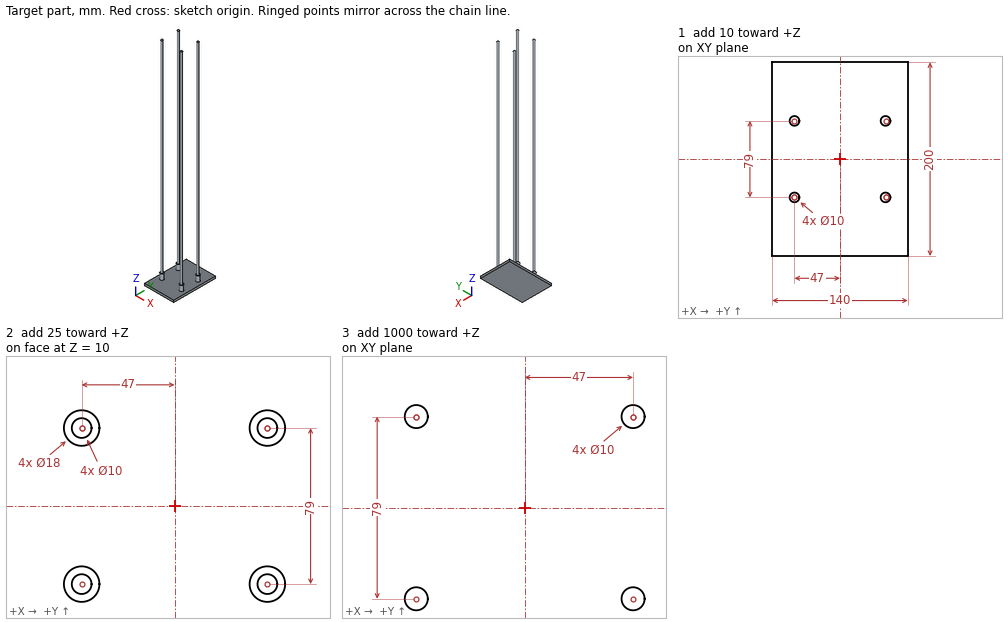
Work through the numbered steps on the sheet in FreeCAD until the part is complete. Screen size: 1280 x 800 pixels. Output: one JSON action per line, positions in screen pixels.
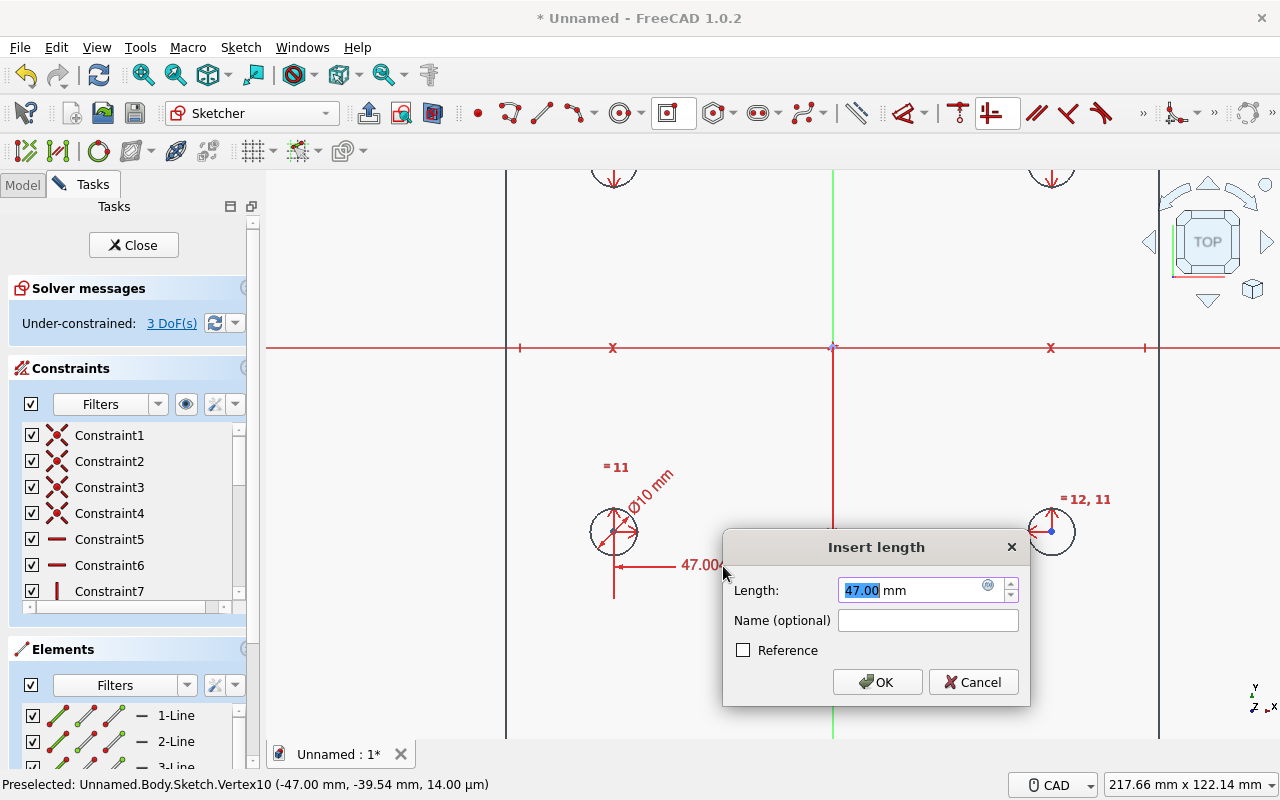
{"action": "type", "text": "47"}
{"action": "key", "text": "Return"}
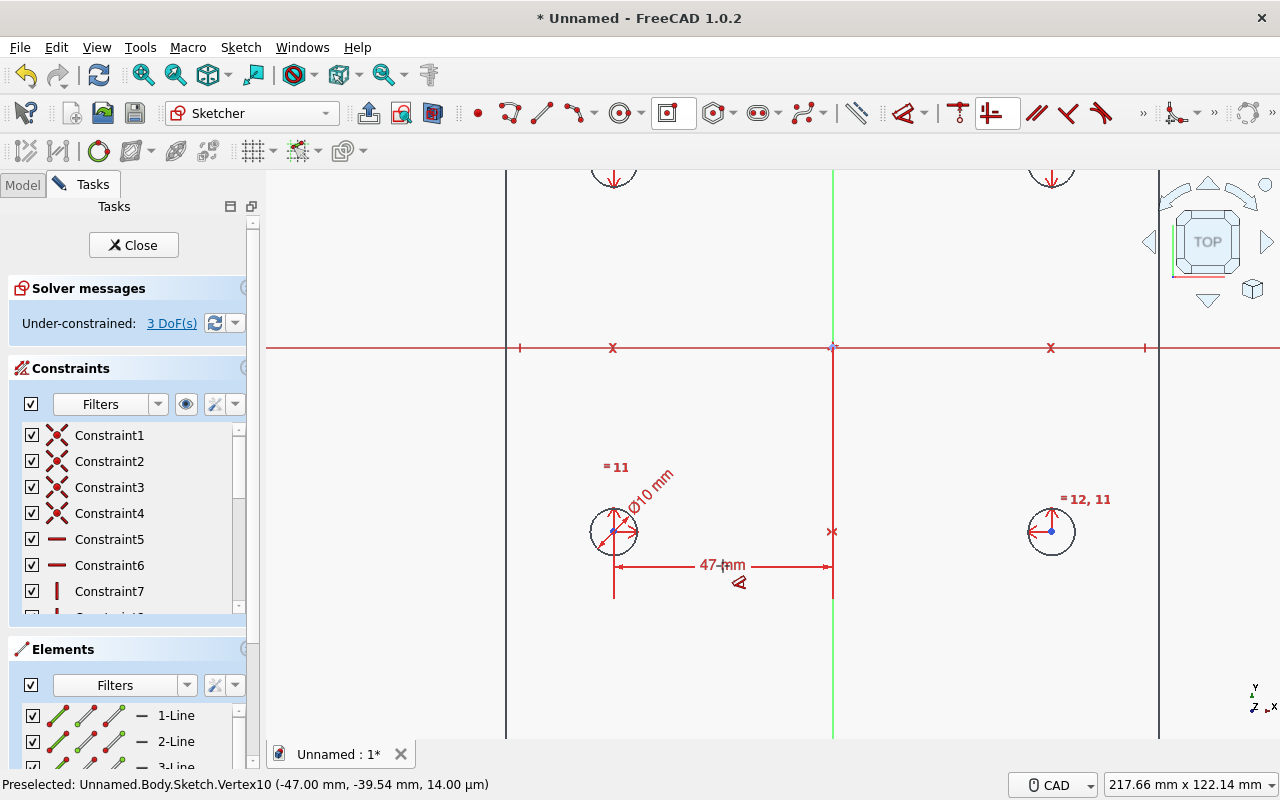
{"action": "scroll", "coordinate": [630, 517], "scroll_direction": "down", "scroll_amount": 5}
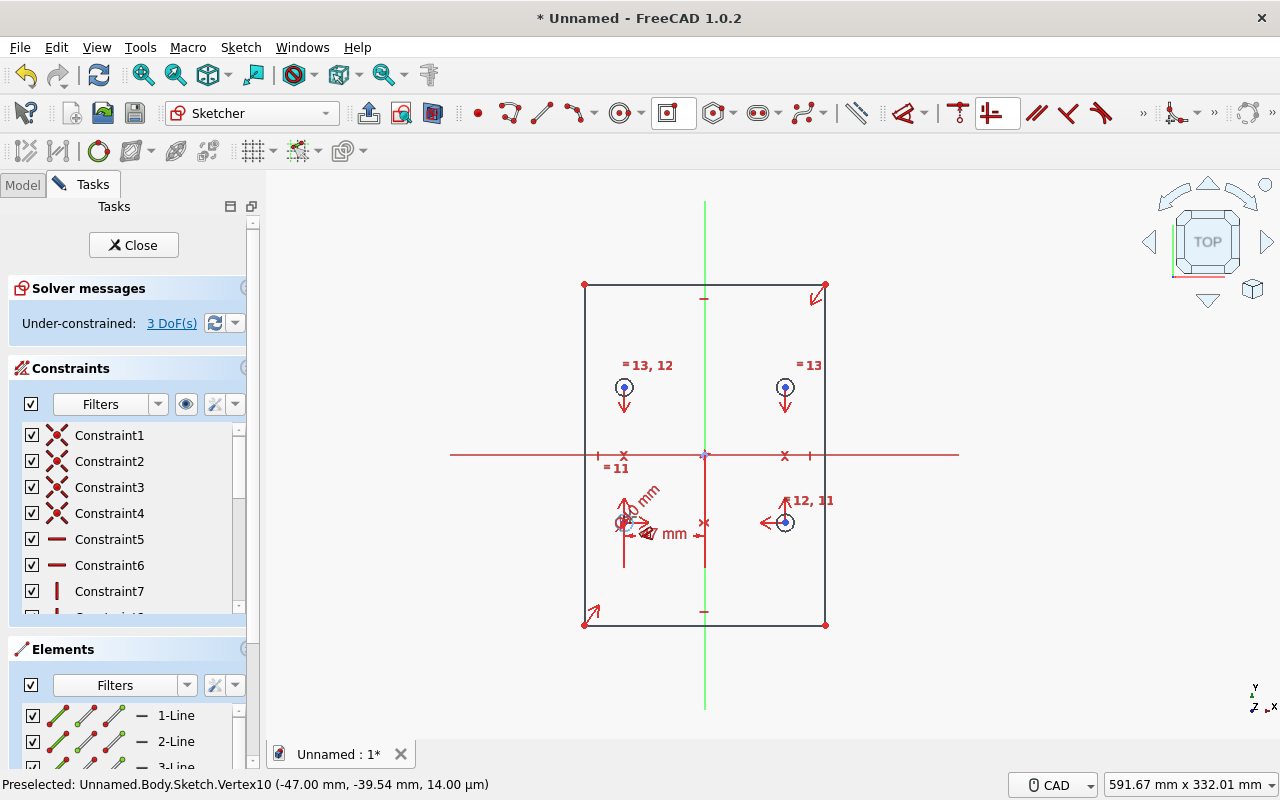
{"action": "left_click", "coordinate": [657, 626]}
{"action": "left_click", "coordinate": [650, 660]}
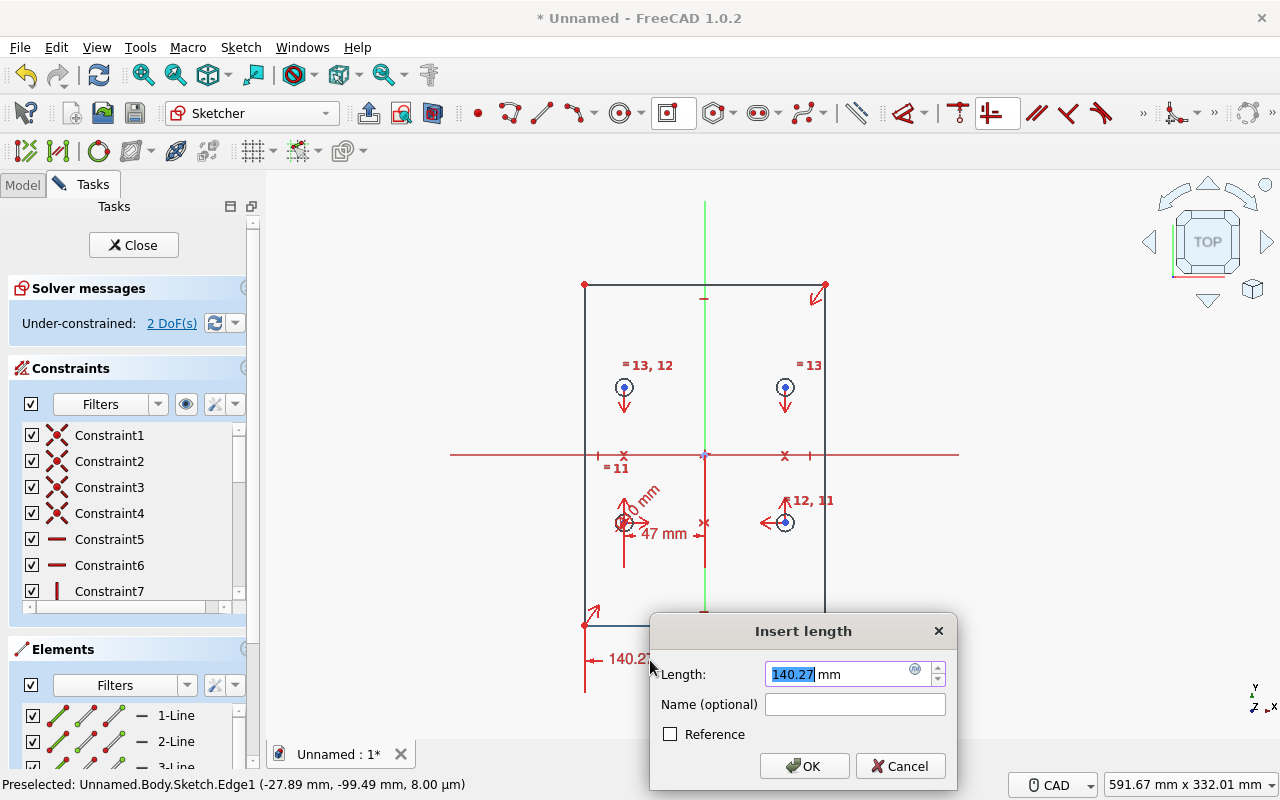
{"action": "type", "text": "140"}
{"action": "key", "text": "Return"}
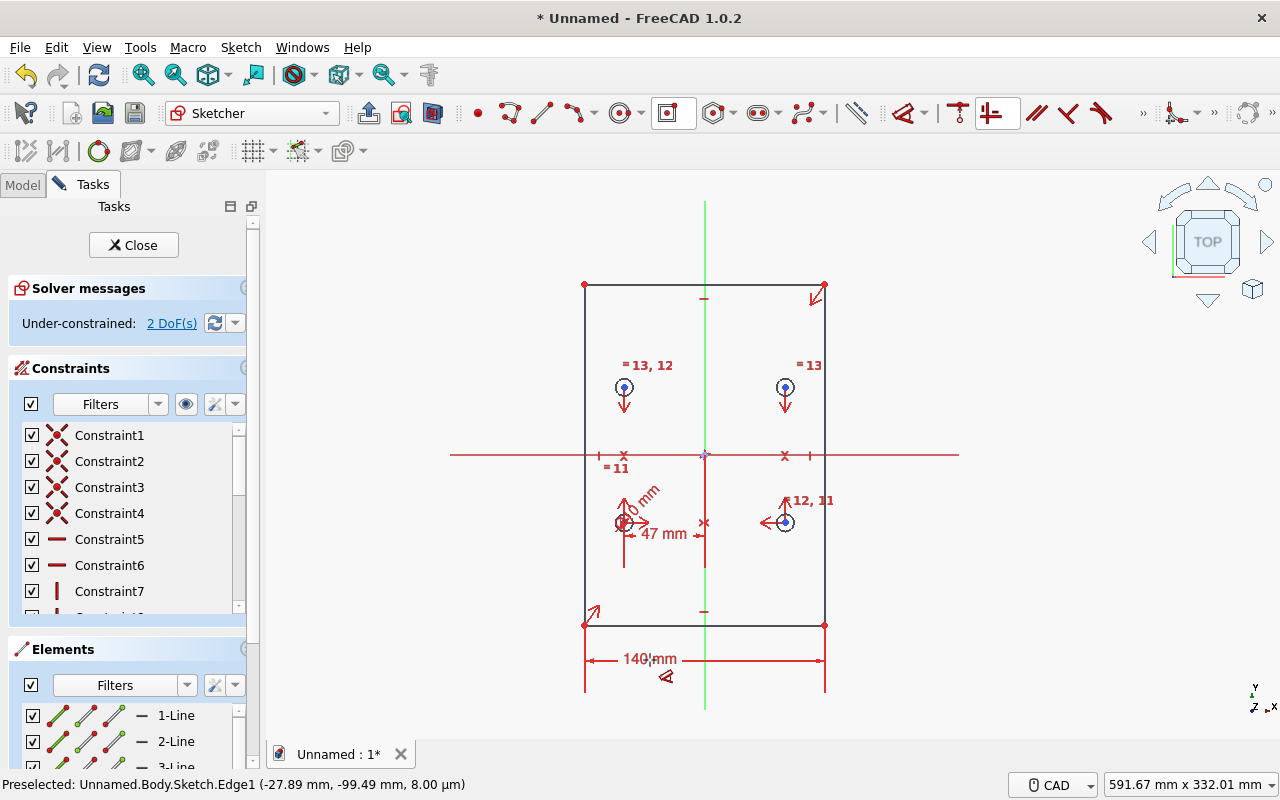
{"action": "left_click", "coordinate": [825, 523]}
{"action": "left_click", "coordinate": [859, 377]}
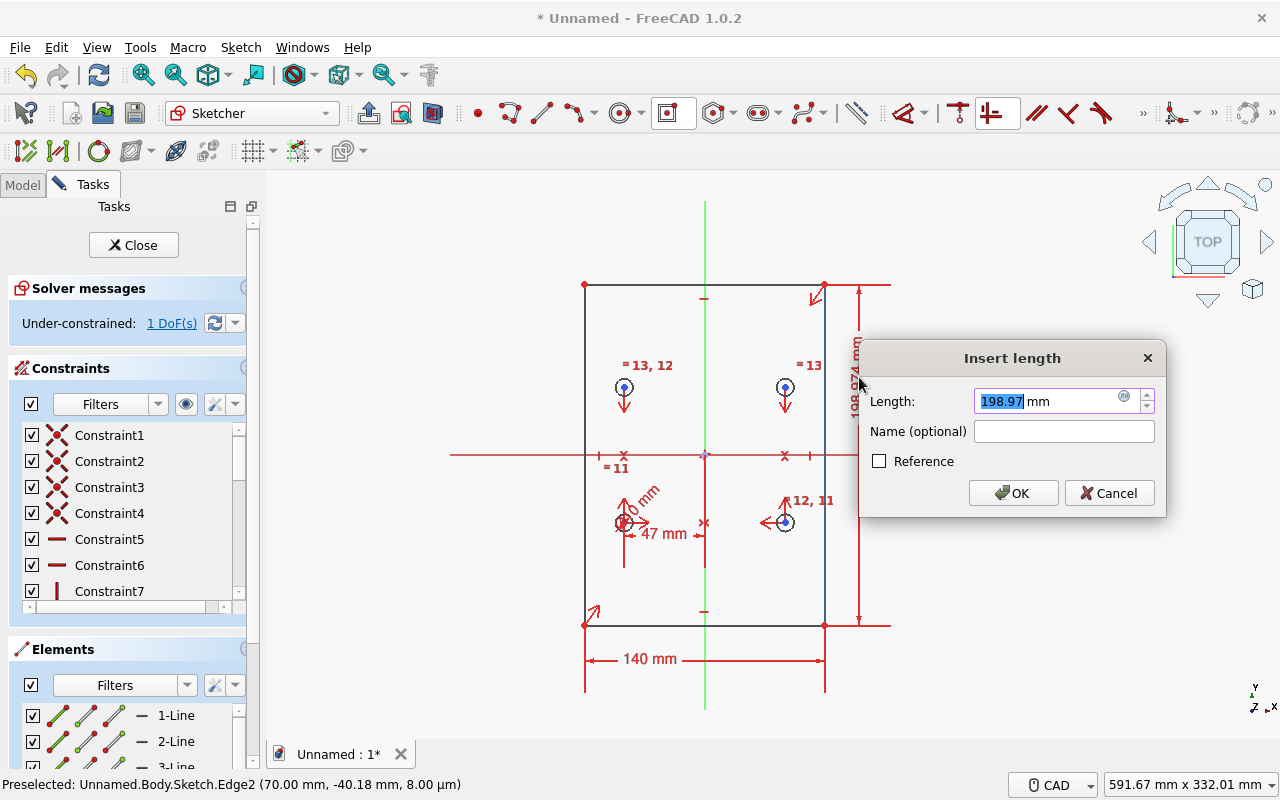
{"action": "type", "text": "200"}
{"action": "key", "text": "Return"}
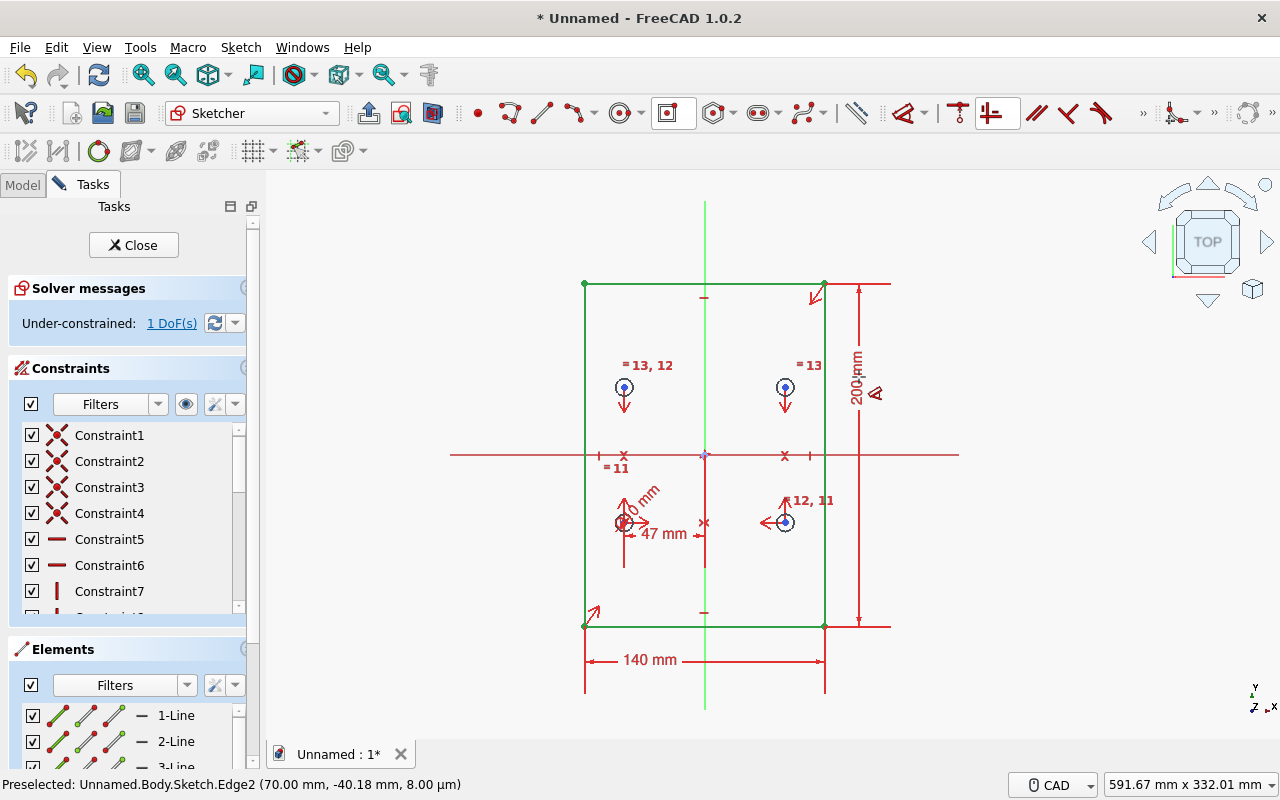
{"action": "left_click", "coordinate": [624, 523]}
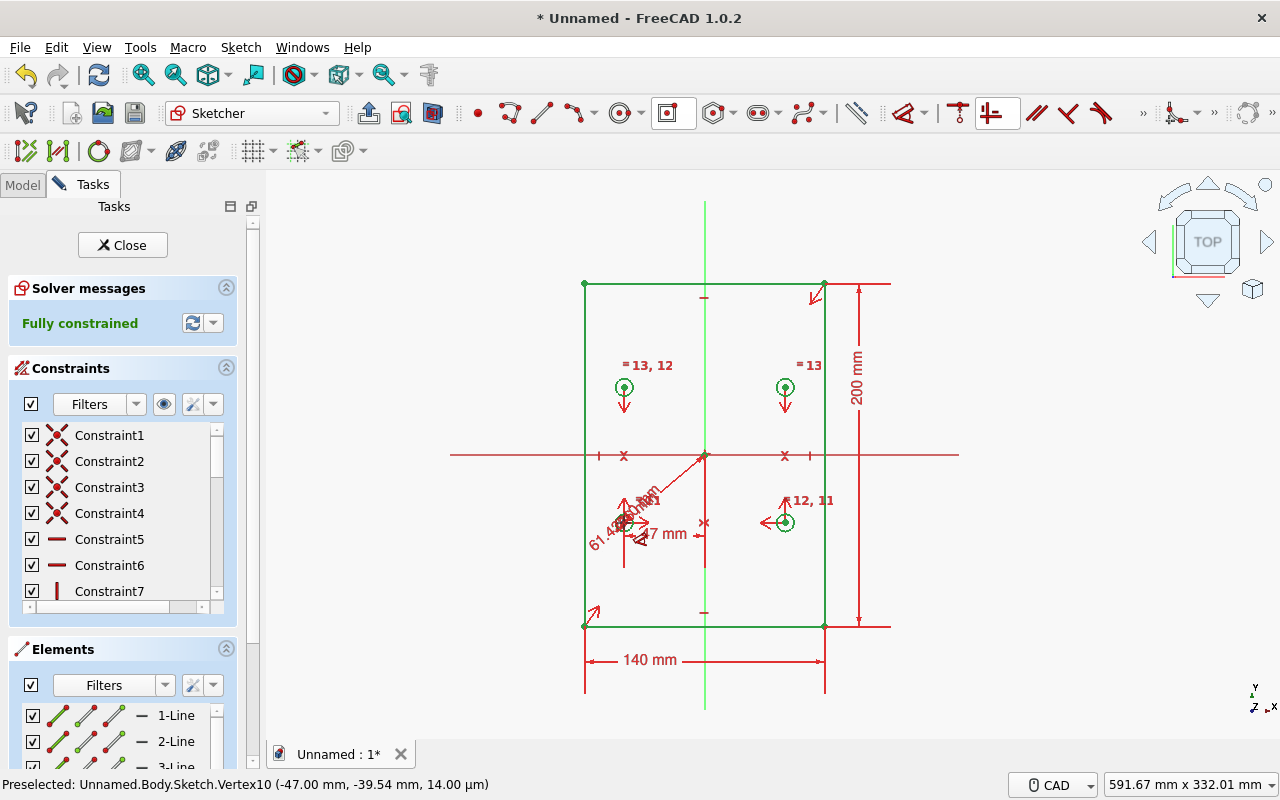
{"action": "left_click", "coordinate": [624, 387]}
{"action": "left_click", "coordinate": [658, 424]}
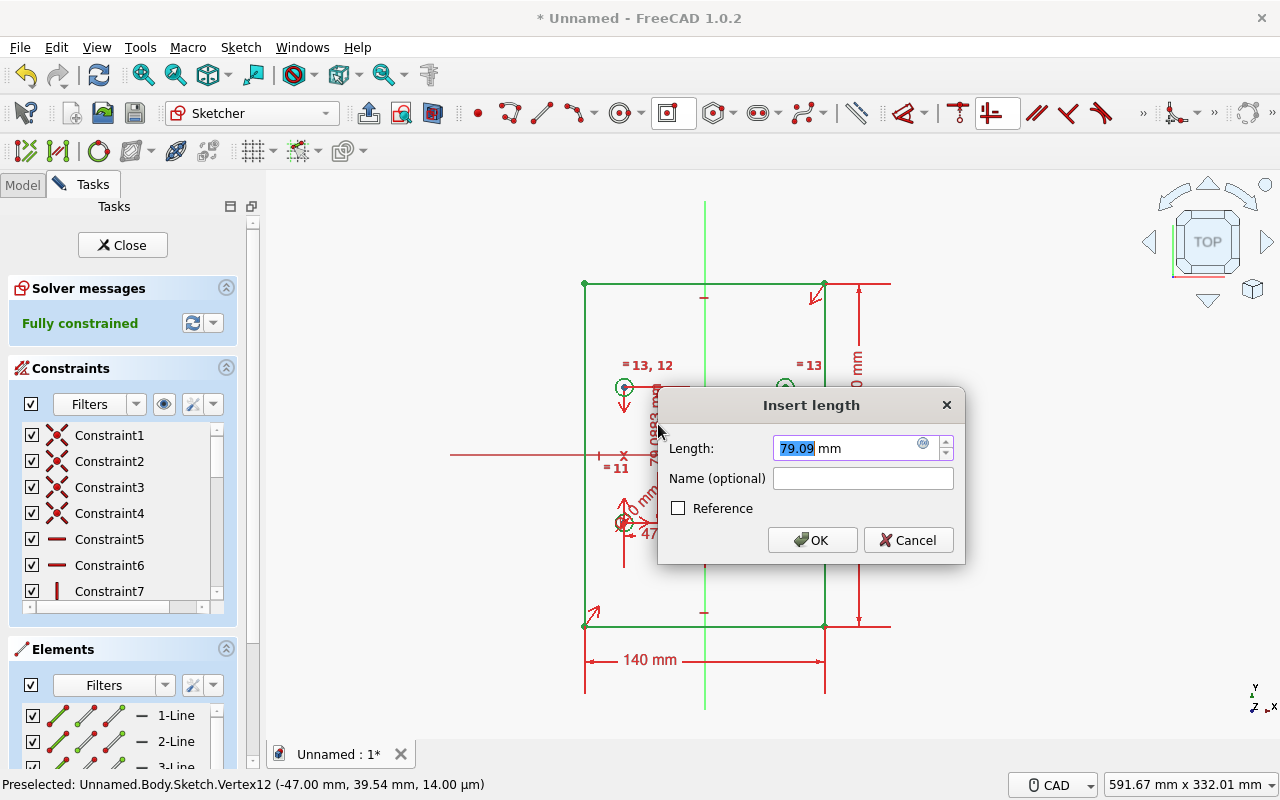
{"action": "type", "text": "79"}
{"action": "key", "text": "Return"}
{"action": "key", "text": "Escape"}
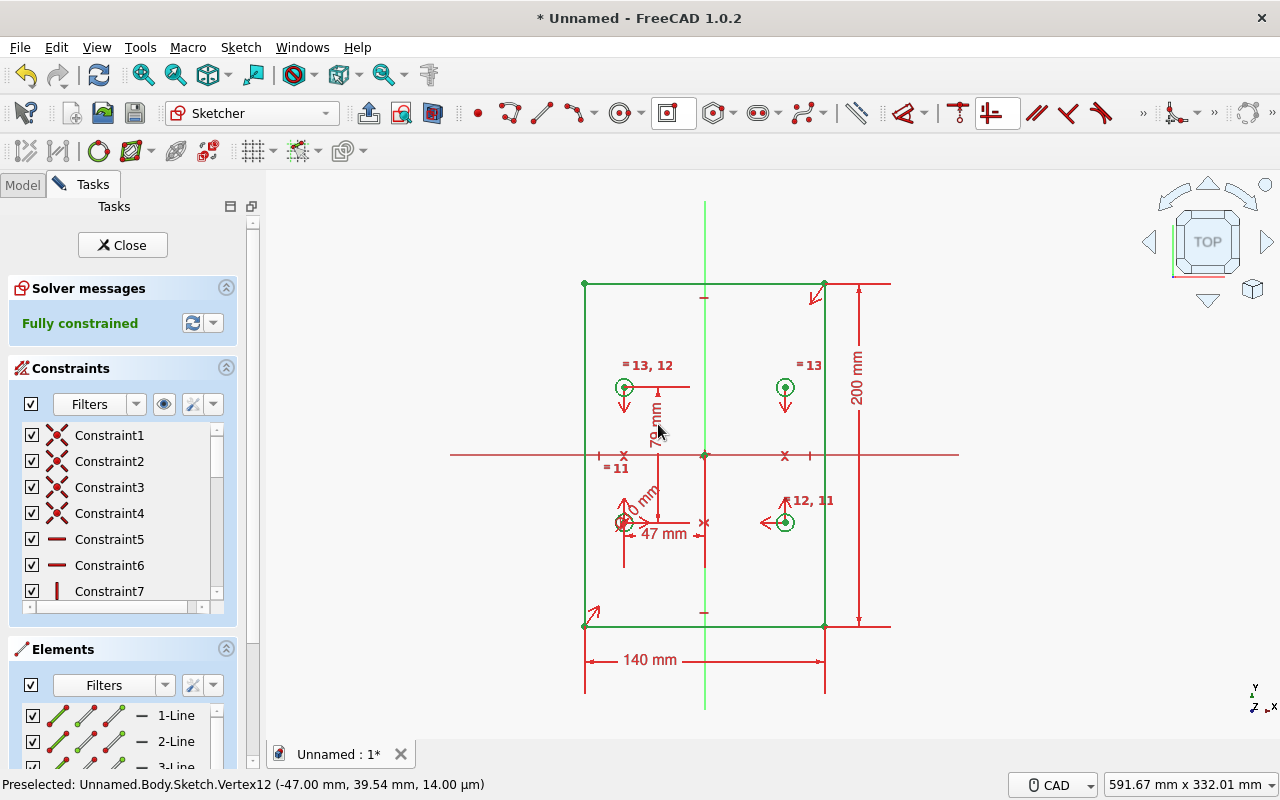
{"action": "left_click", "coordinate": [123, 245]}